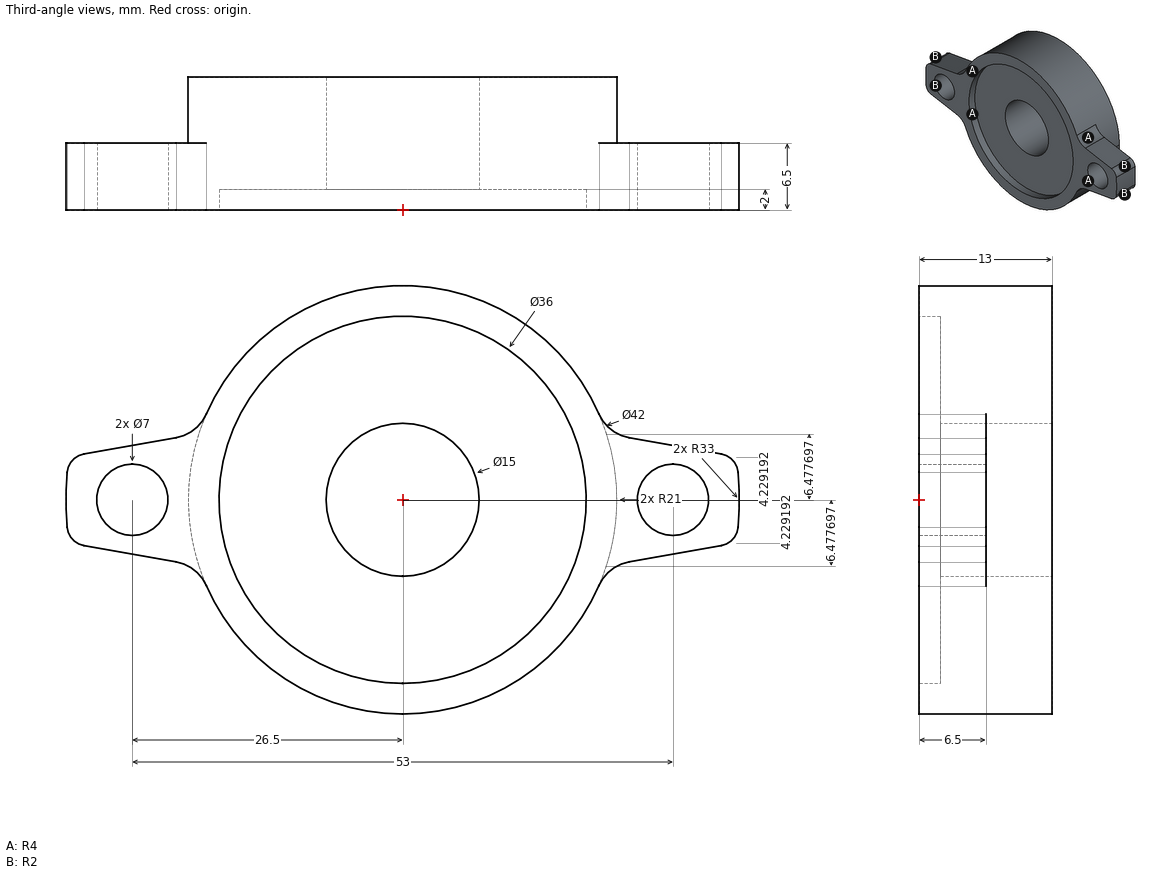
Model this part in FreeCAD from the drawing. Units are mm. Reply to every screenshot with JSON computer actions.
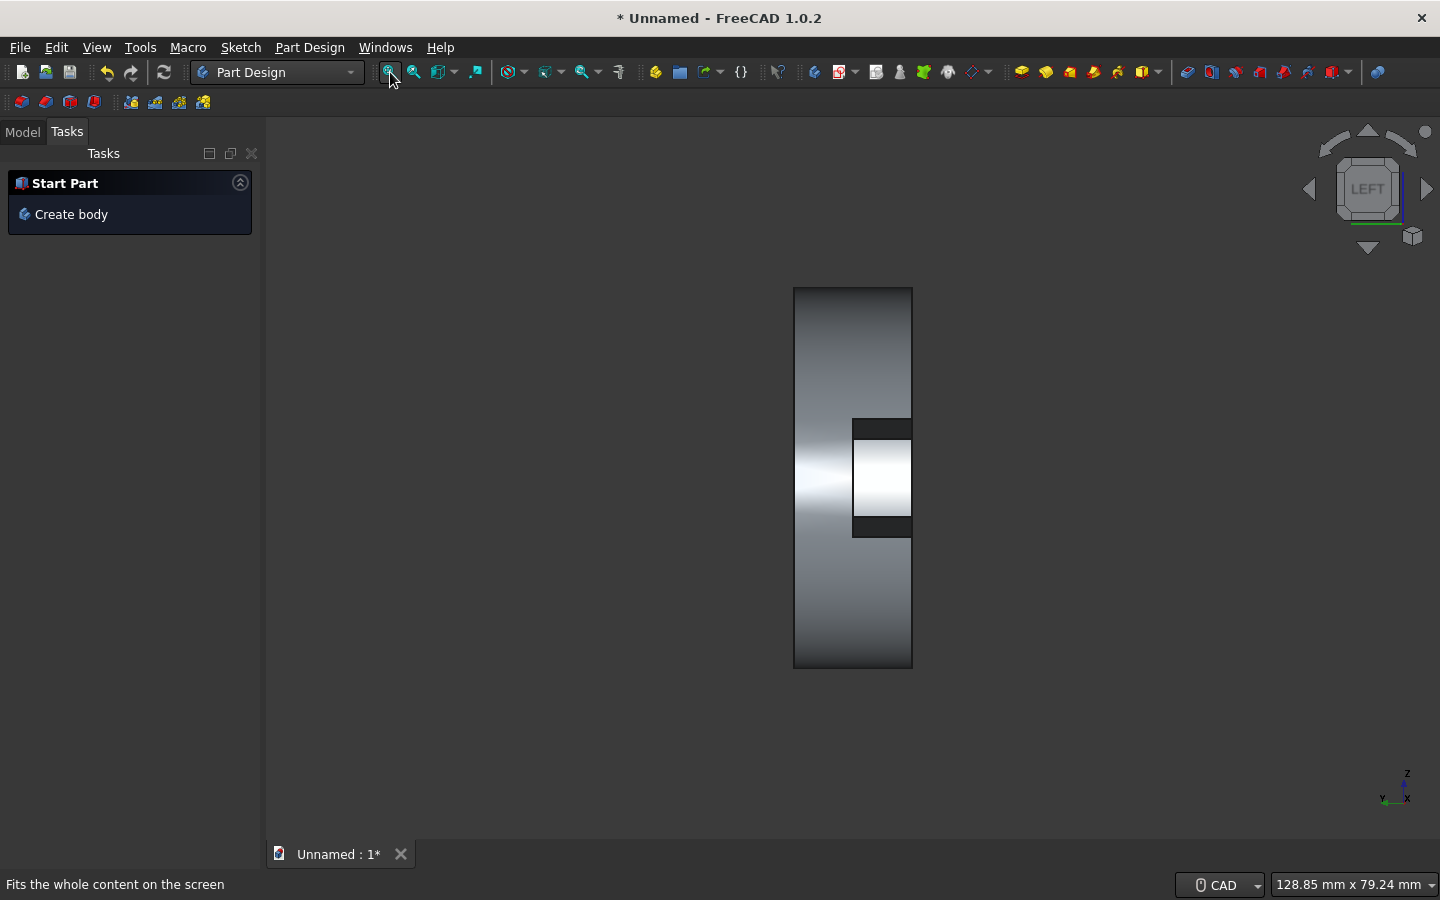
{"action": "key", "text": "v 3"}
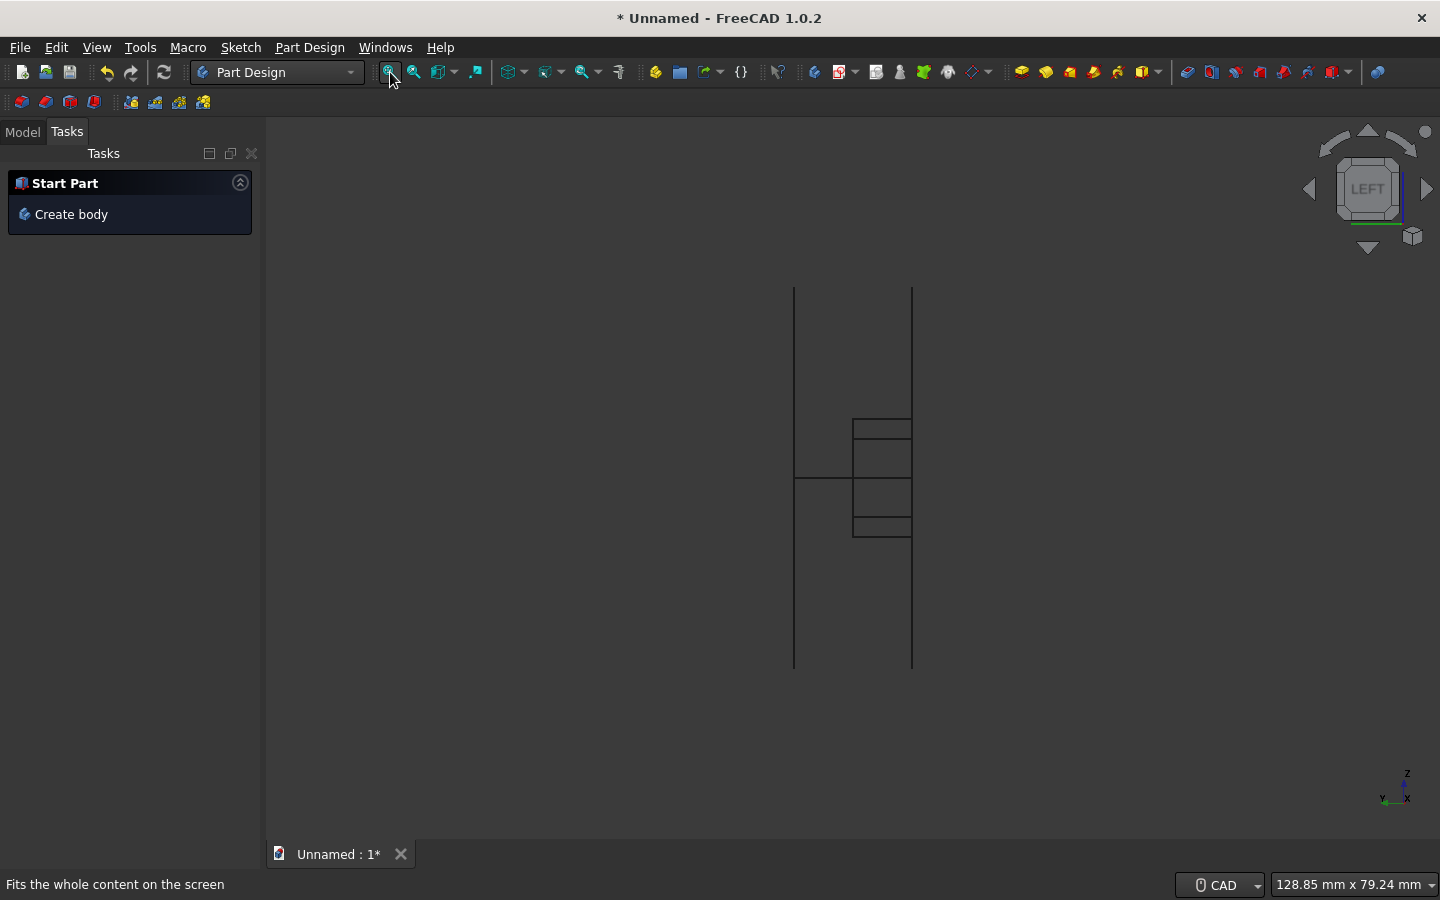
{"action": "key", "text": "0"}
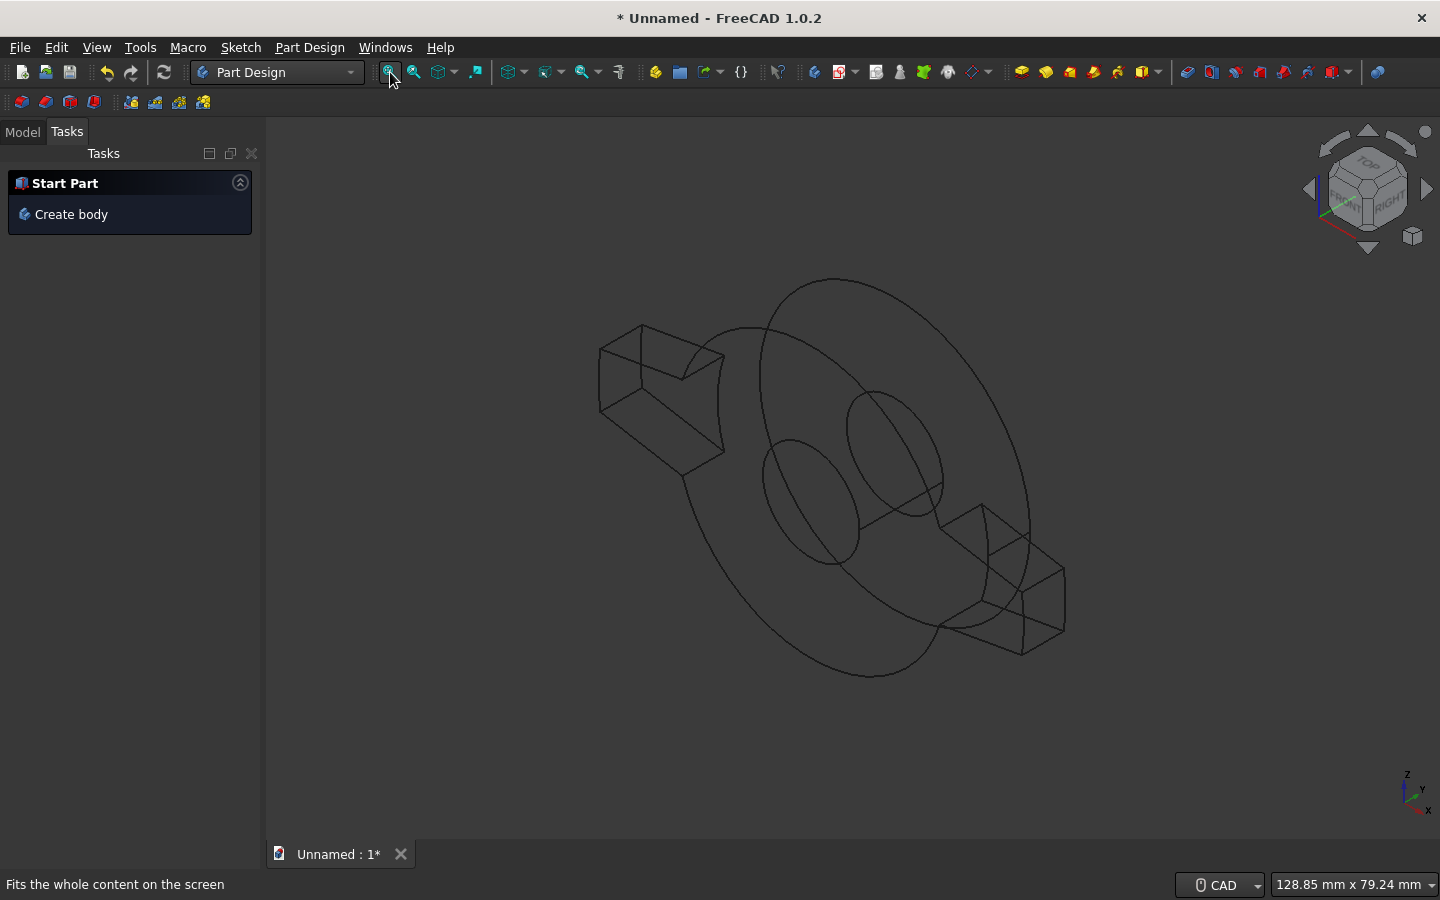
{"action": "left_click", "coordinate": [961, 612]}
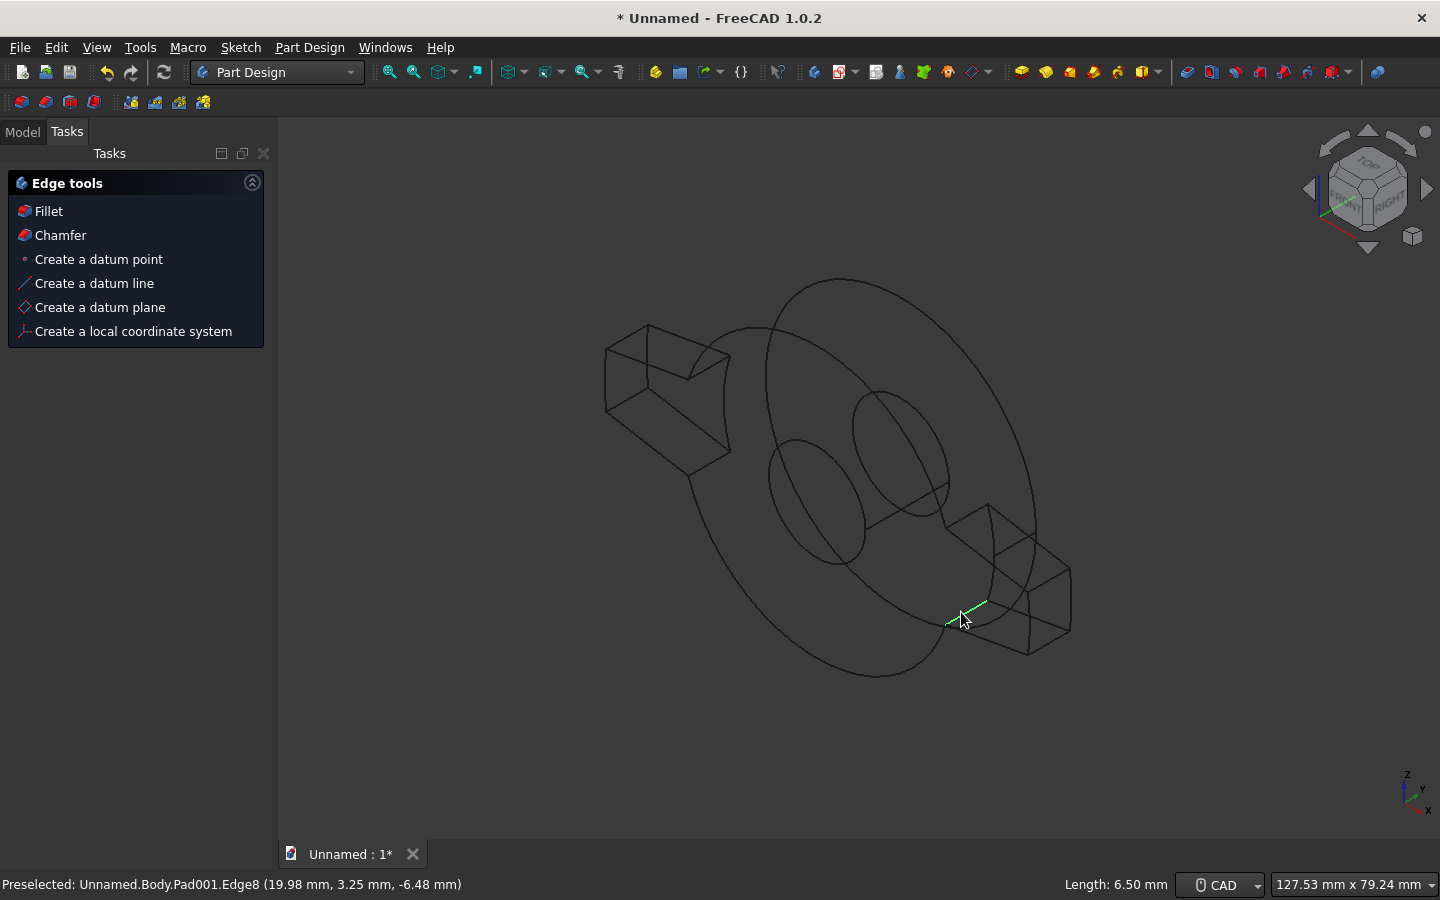
{"action": "left_click", "coordinate": [967, 515], "text": "ctrl"}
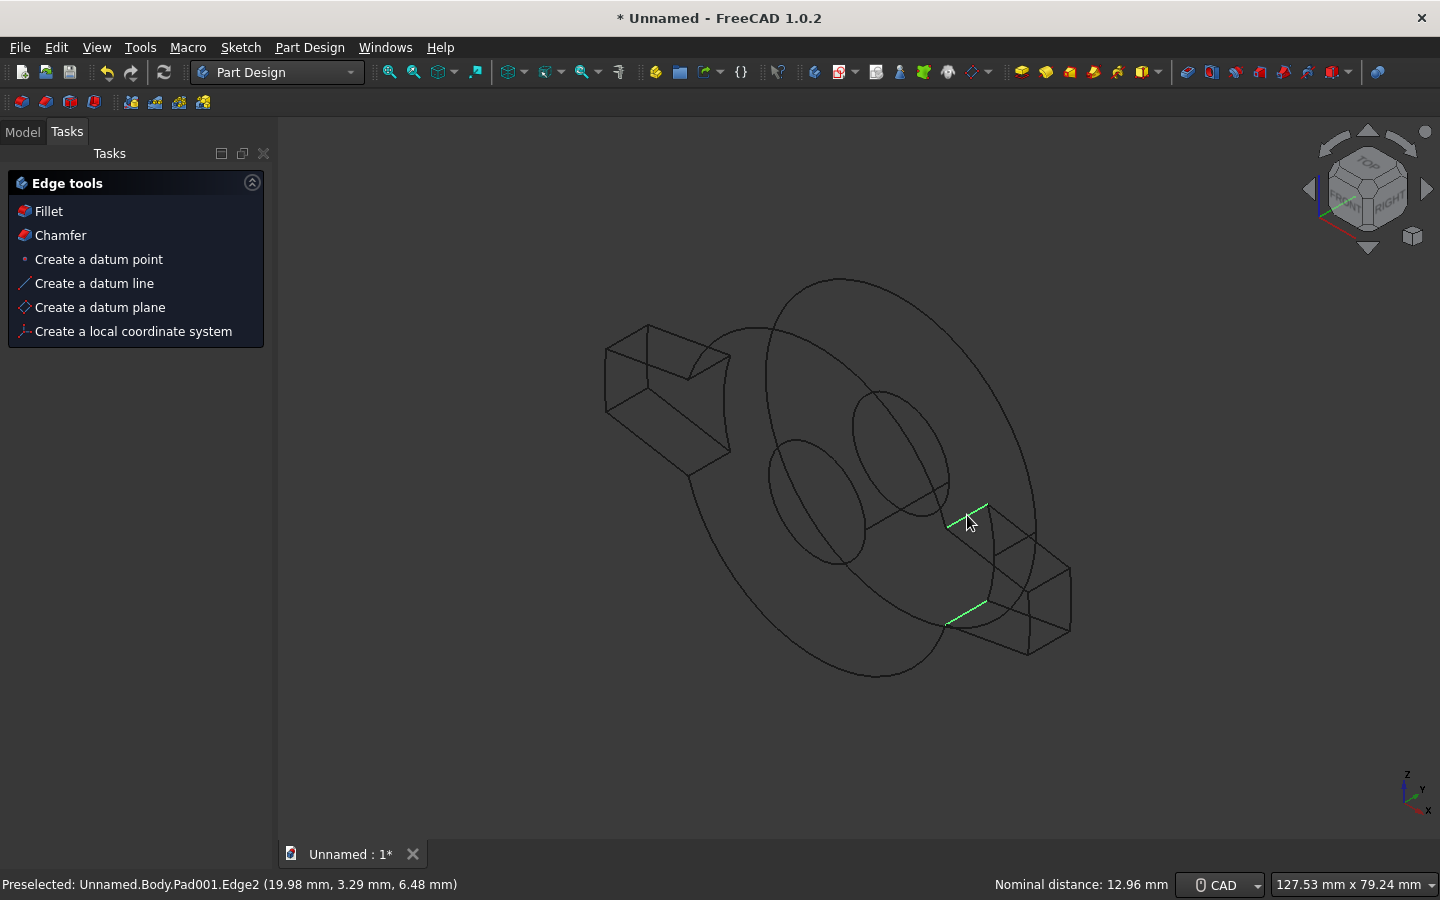
{"action": "left_click", "coordinate": [709, 367], "text": "ctrl"}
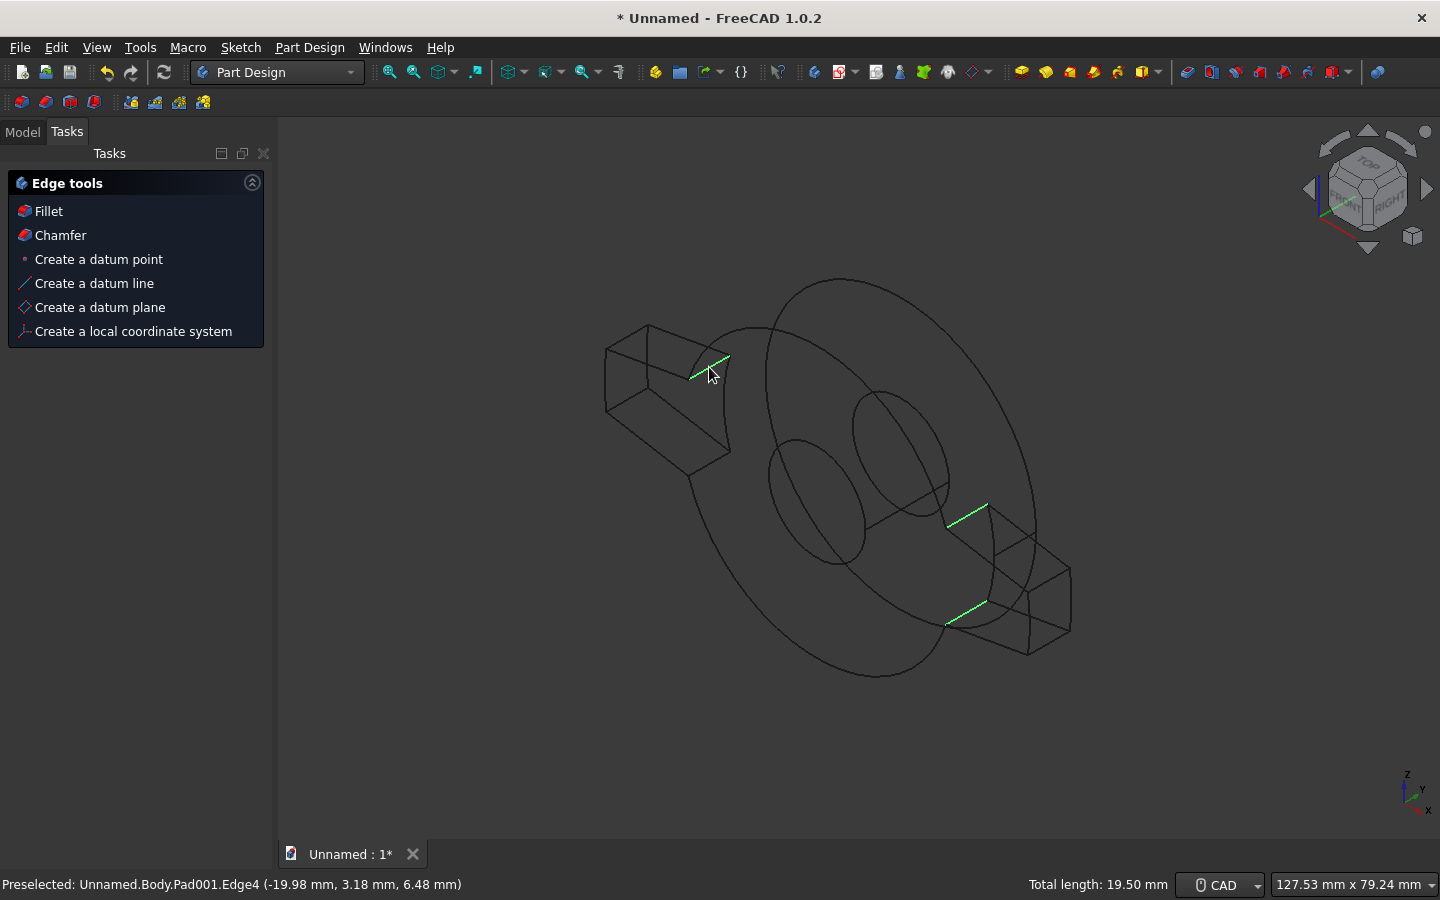
{"action": "left_click", "coordinate": [709, 463], "text": "ctrl"}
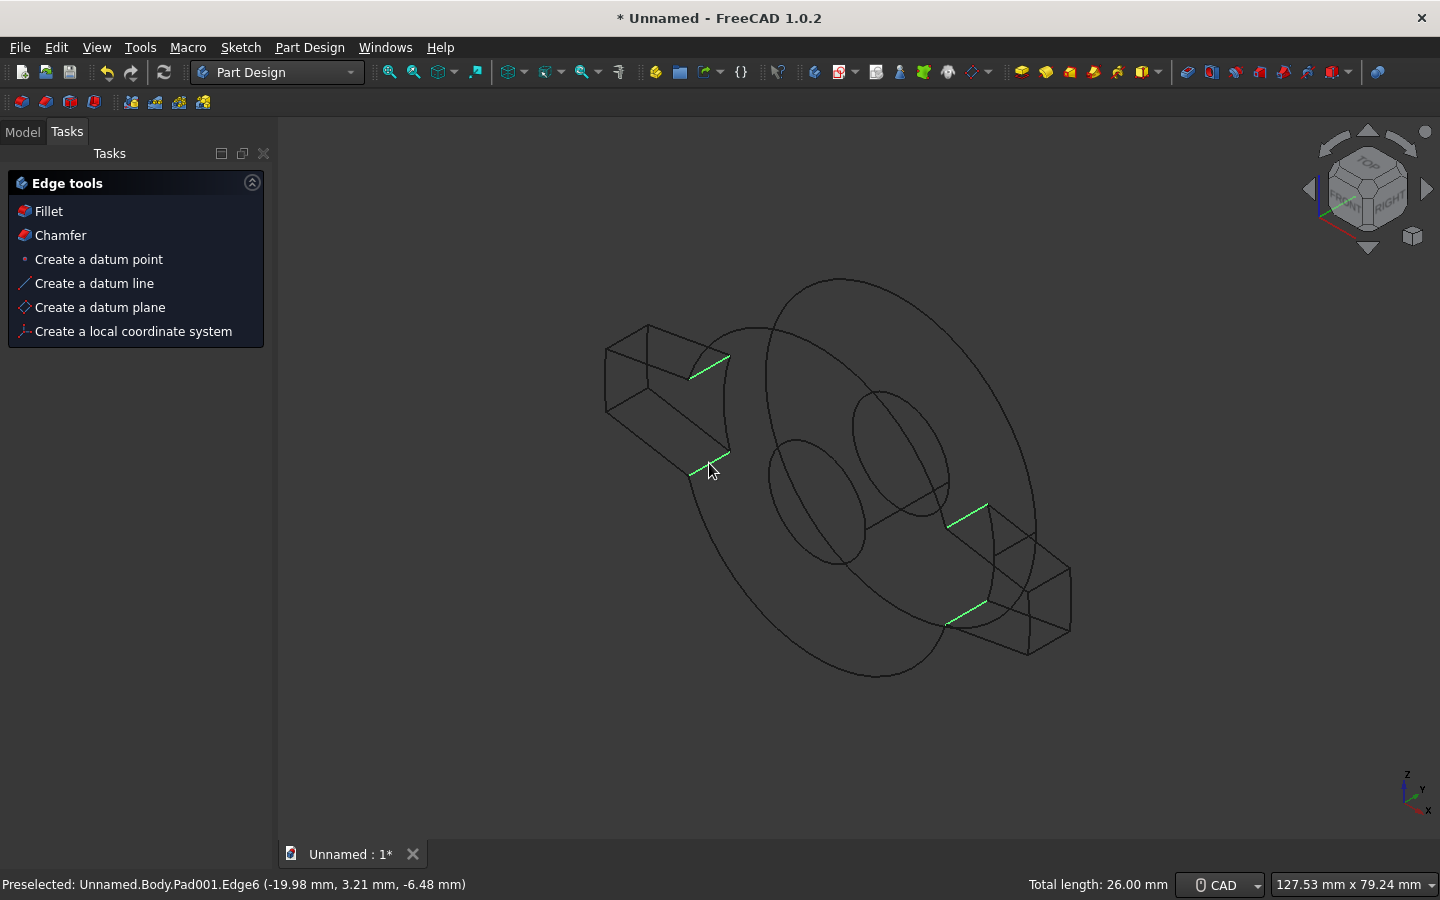
{"action": "key", "text": "v 1"}